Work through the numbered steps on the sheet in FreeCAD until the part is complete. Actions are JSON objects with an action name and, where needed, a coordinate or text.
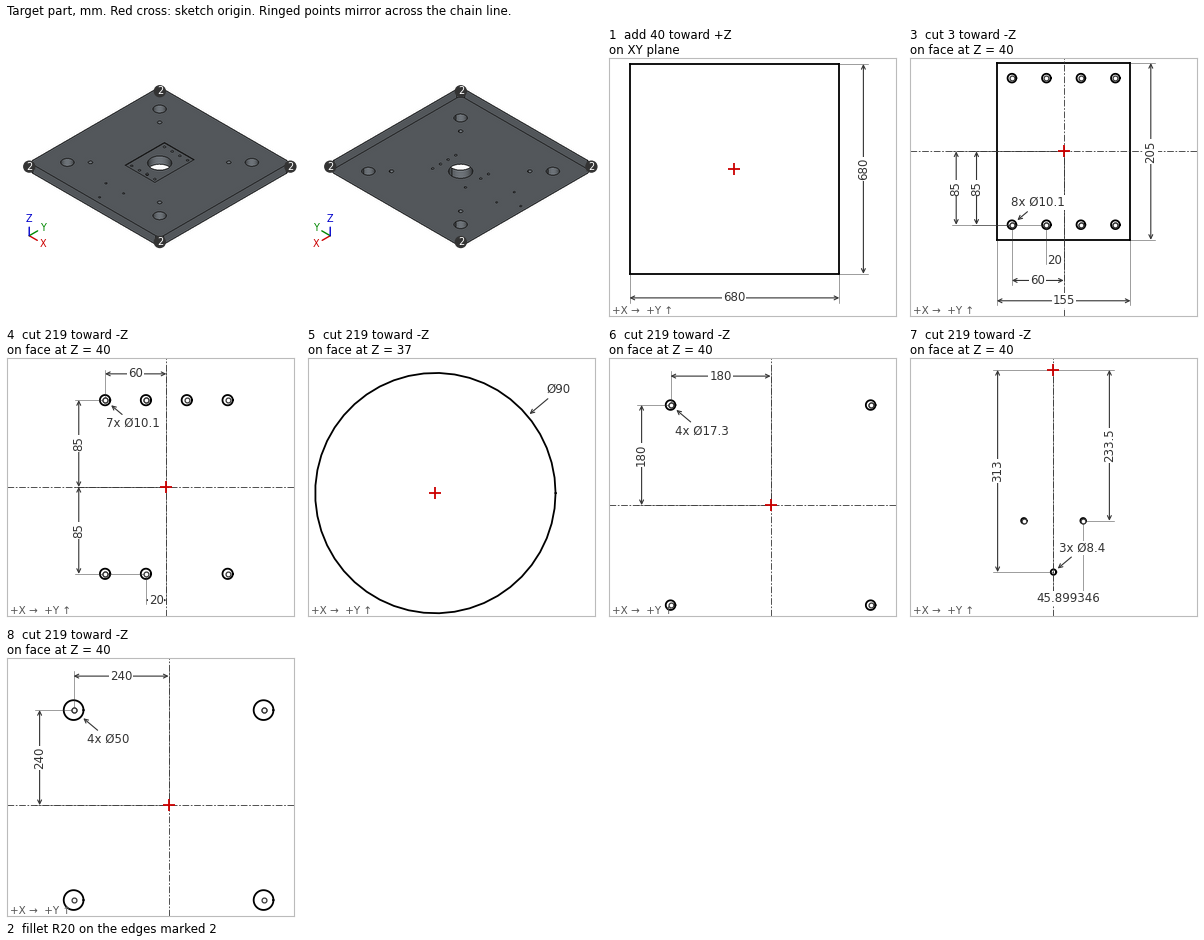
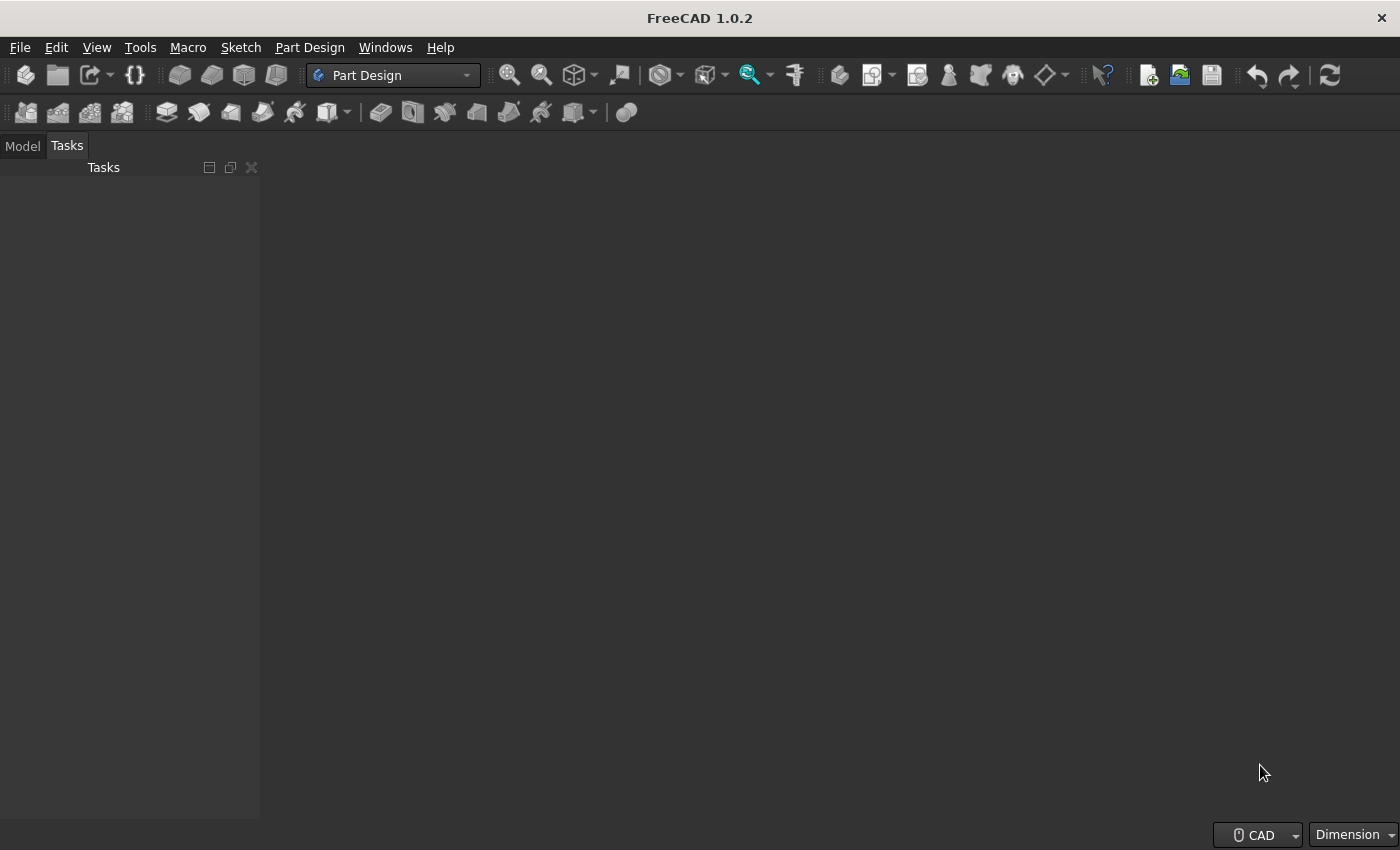
{"action": "left_click", "coordinate": [1148, 76]}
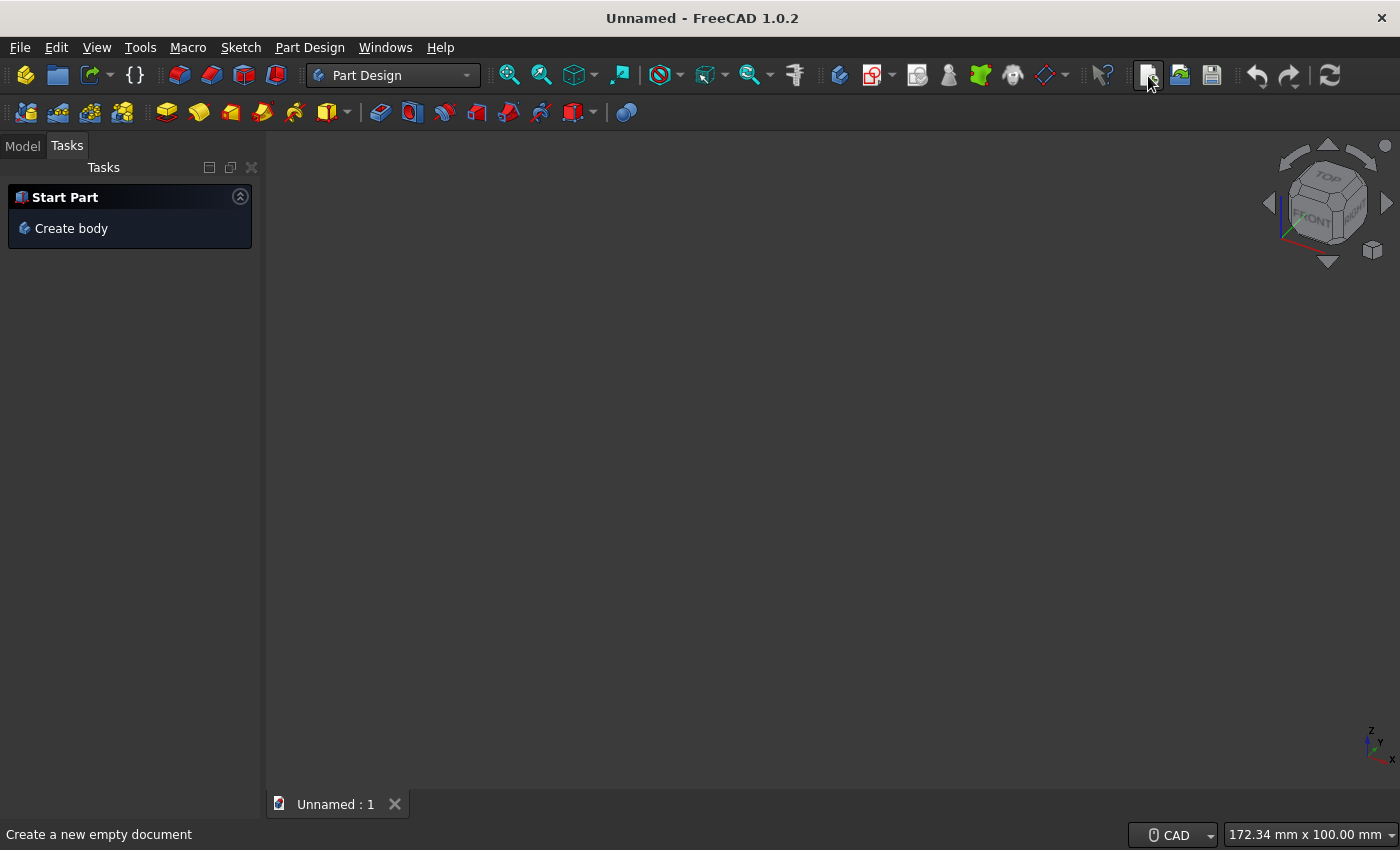
{"action": "left_click", "coordinate": [872, 76]}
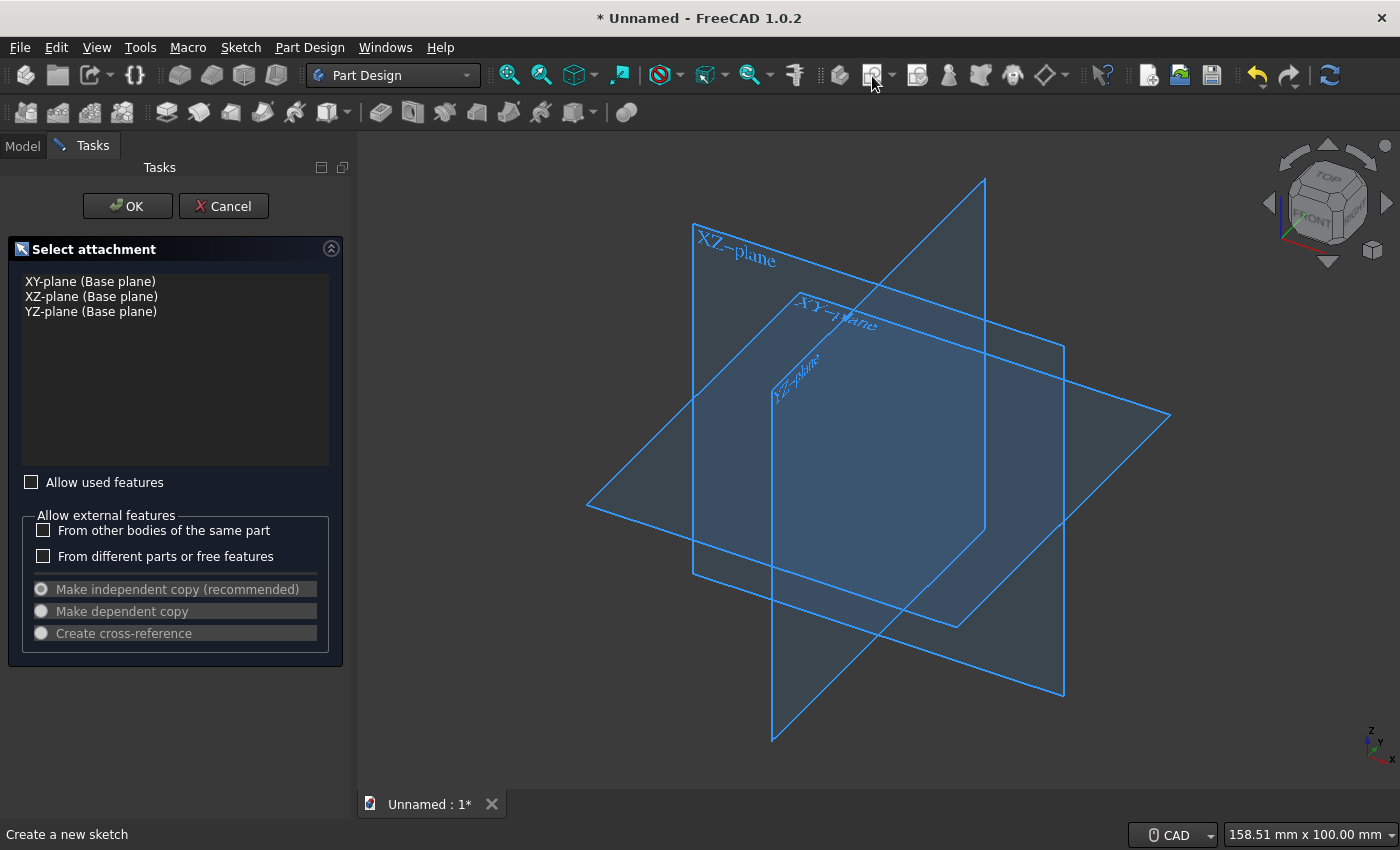
{"action": "left_click", "coordinate": [82, 282]}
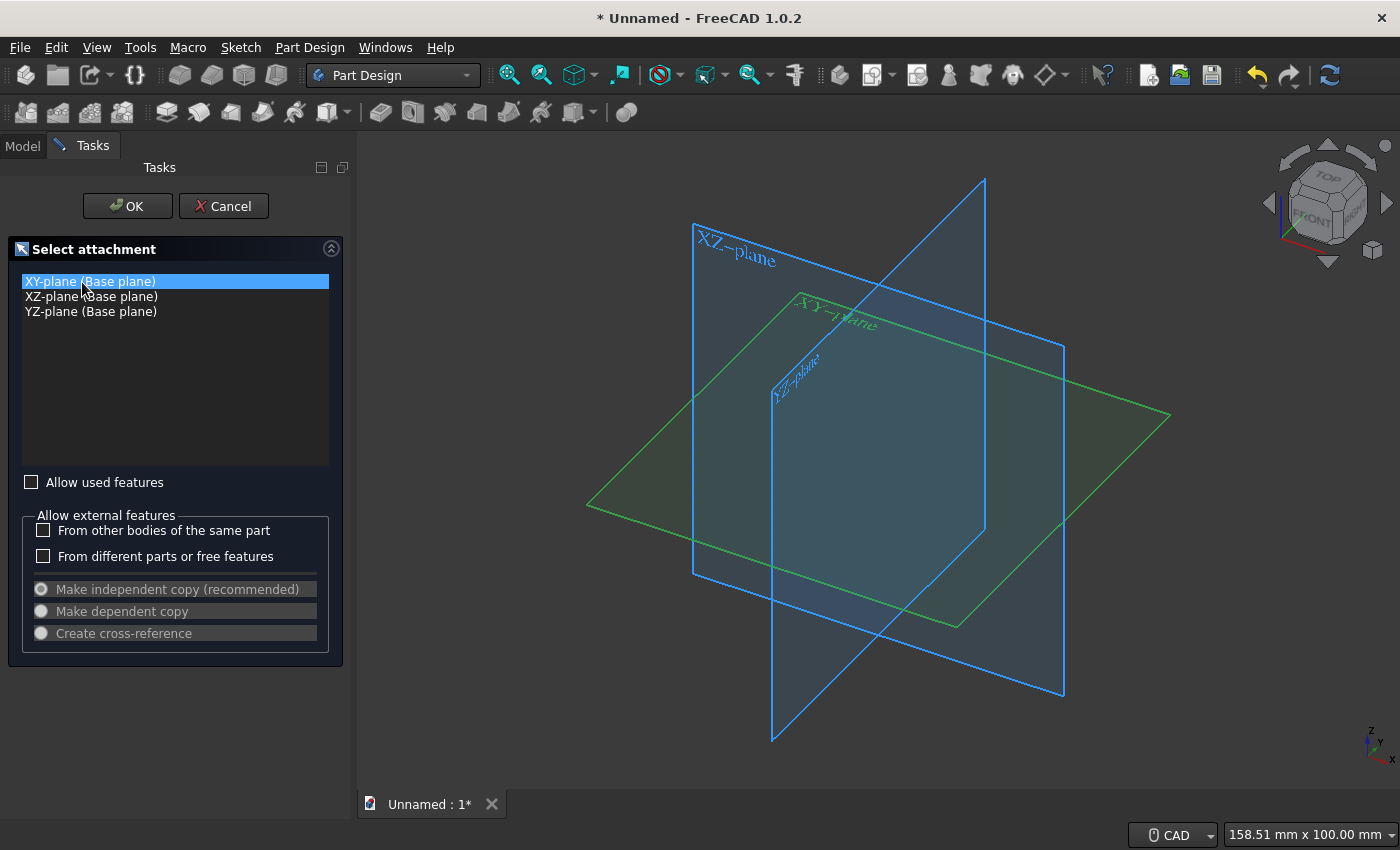
{"action": "left_click", "coordinate": [128, 206]}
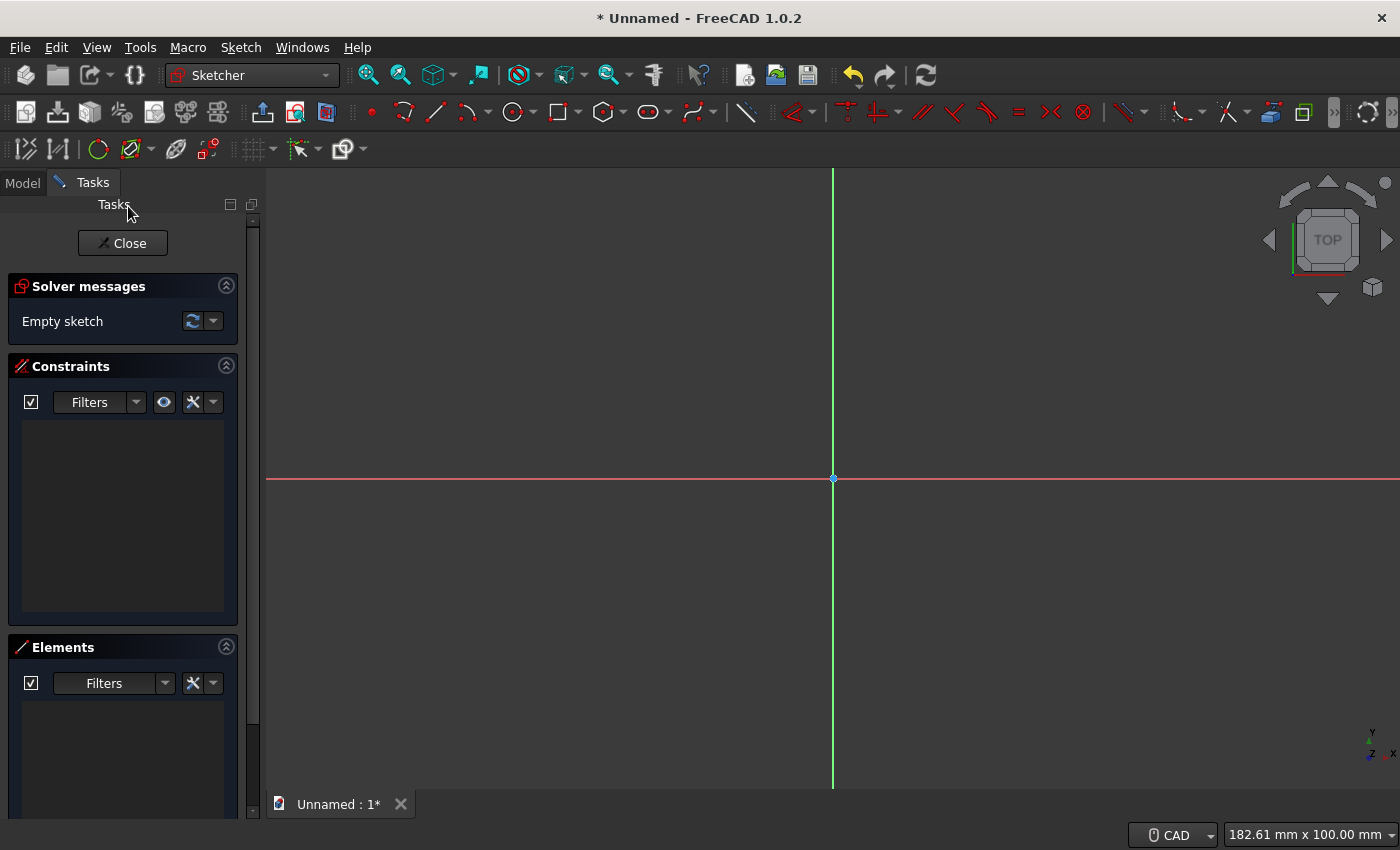
{"action": "scroll", "coordinate": [758, 478], "scroll_direction": "down", "scroll_amount": 12}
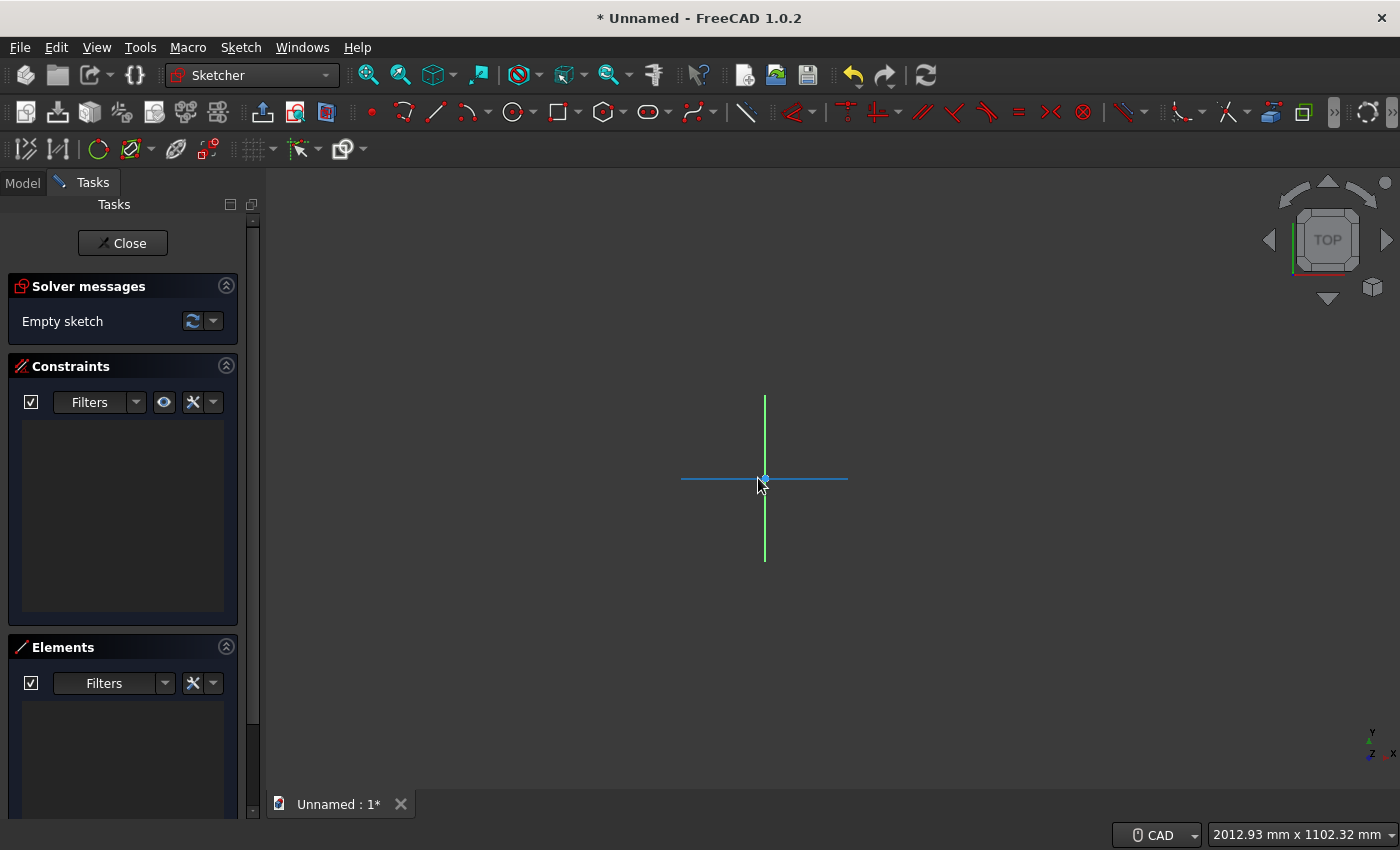
{"action": "key", "text": "g v"}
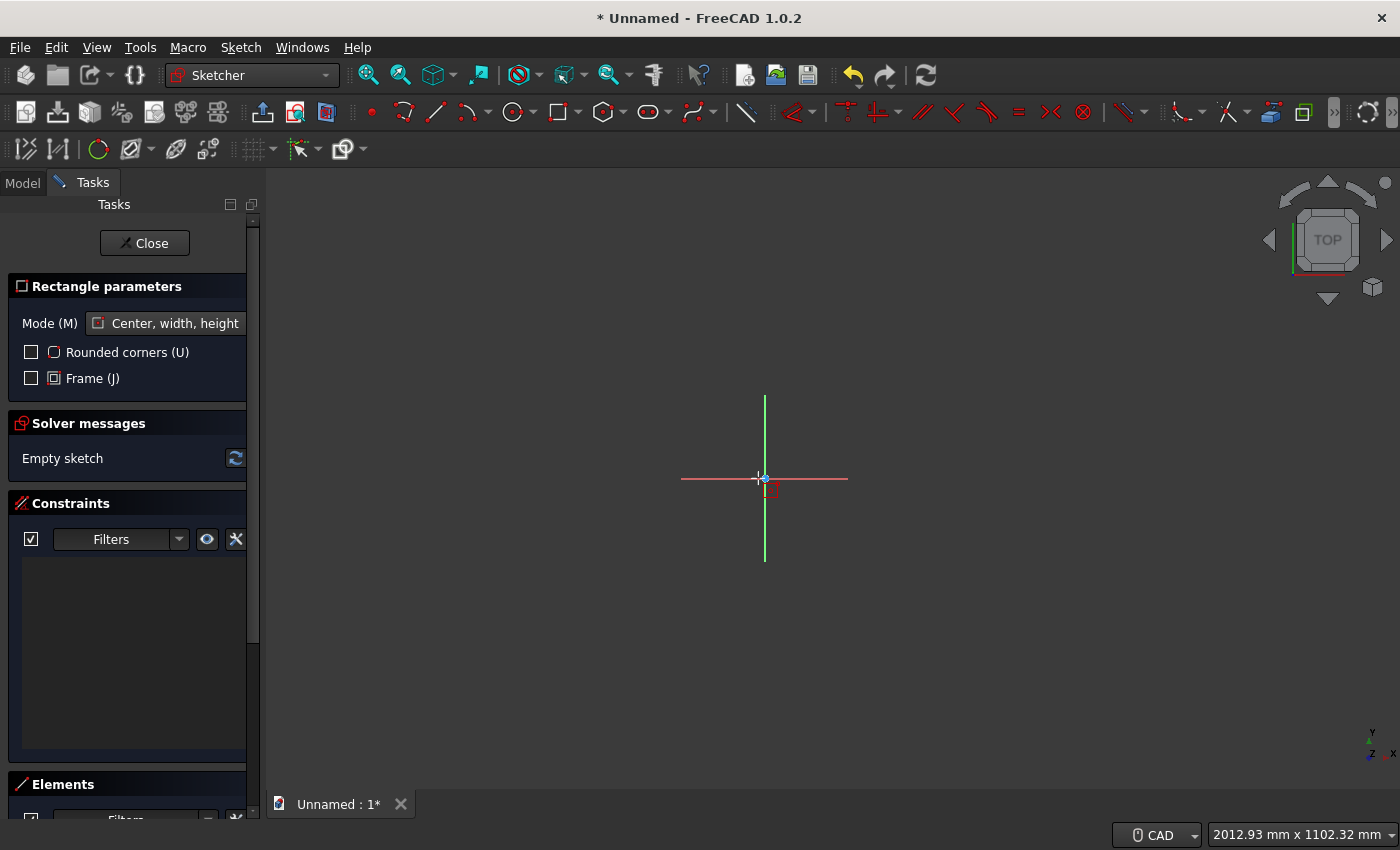
{"action": "left_click", "coordinate": [765, 478]}
{"action": "left_click", "coordinate": [957, 287]}
{"action": "key", "text": "Escape"}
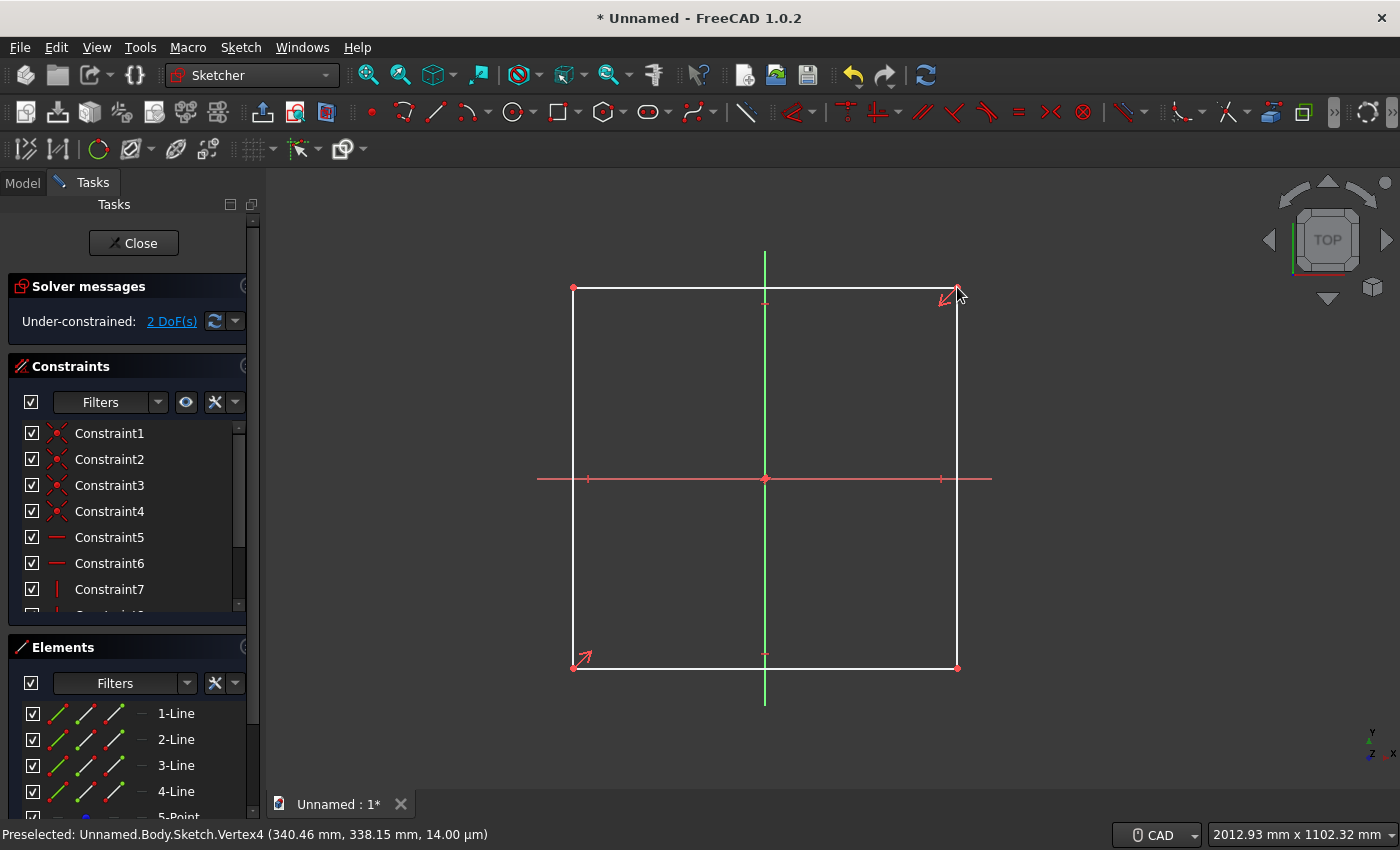
{"action": "left_click", "coordinate": [792, 112]}